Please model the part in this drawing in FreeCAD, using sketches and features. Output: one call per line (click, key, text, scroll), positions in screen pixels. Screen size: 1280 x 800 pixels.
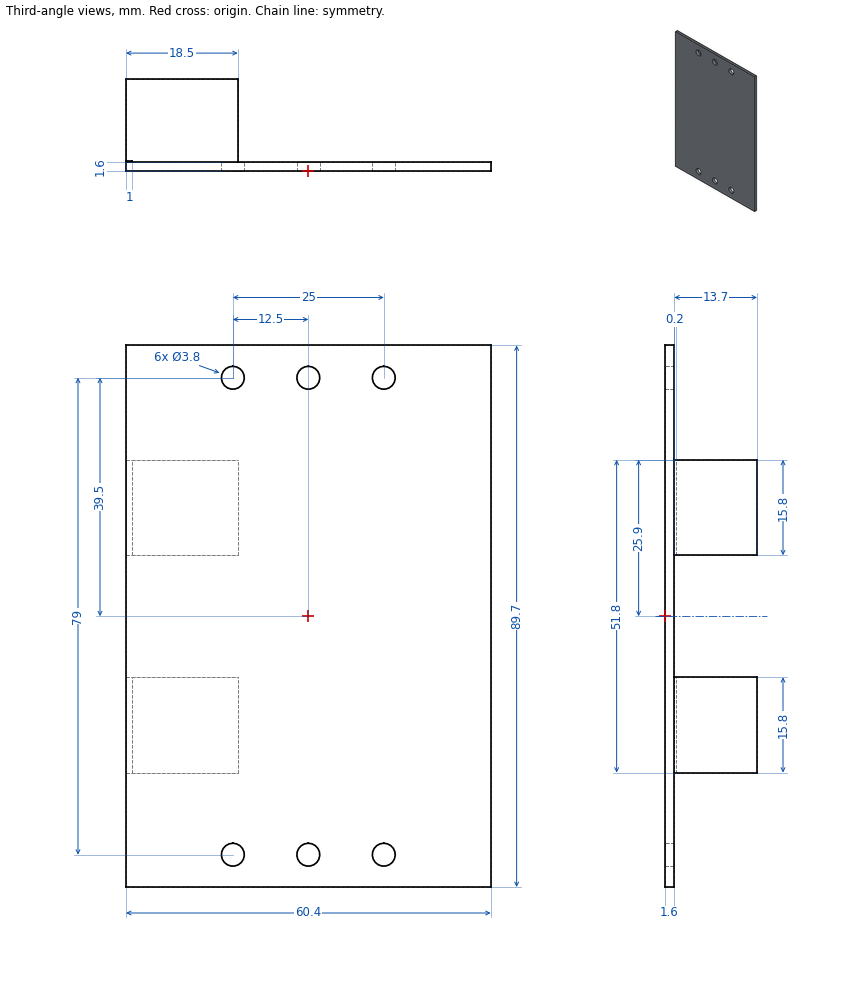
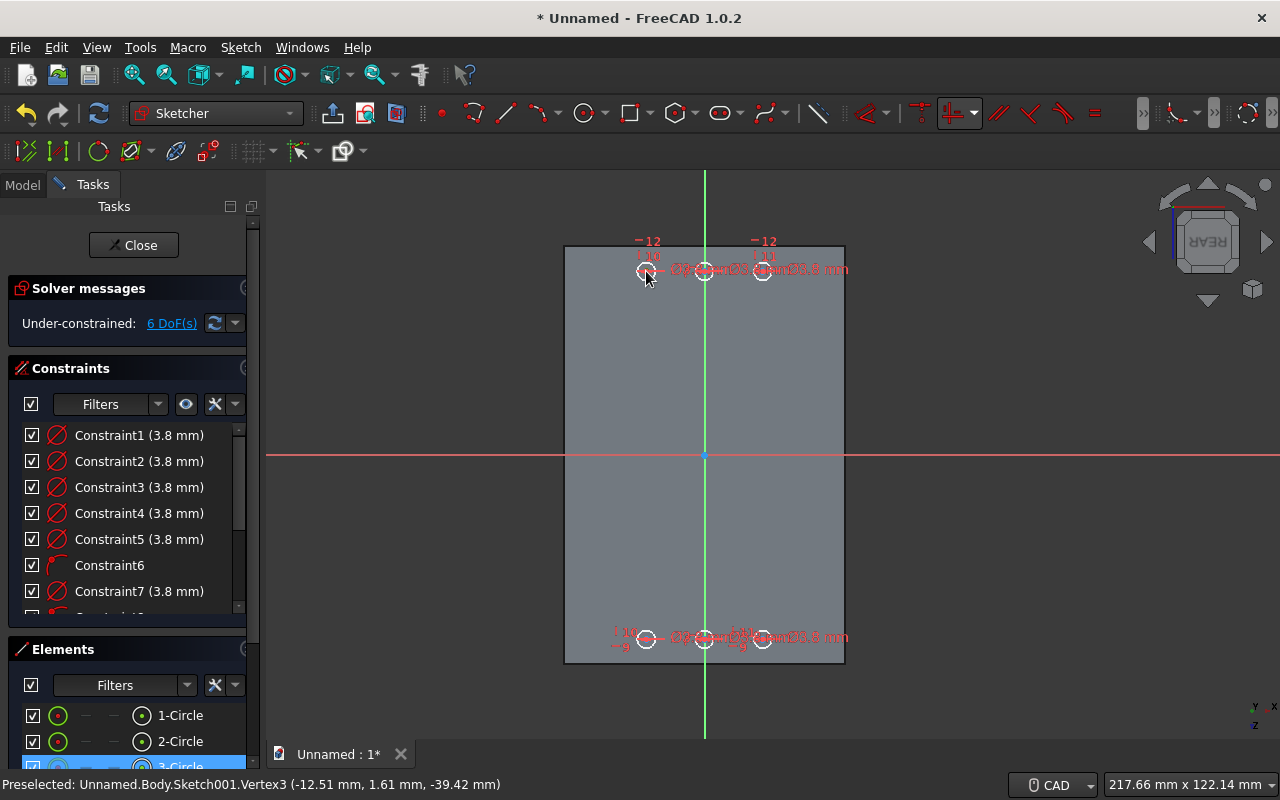
click(705, 271)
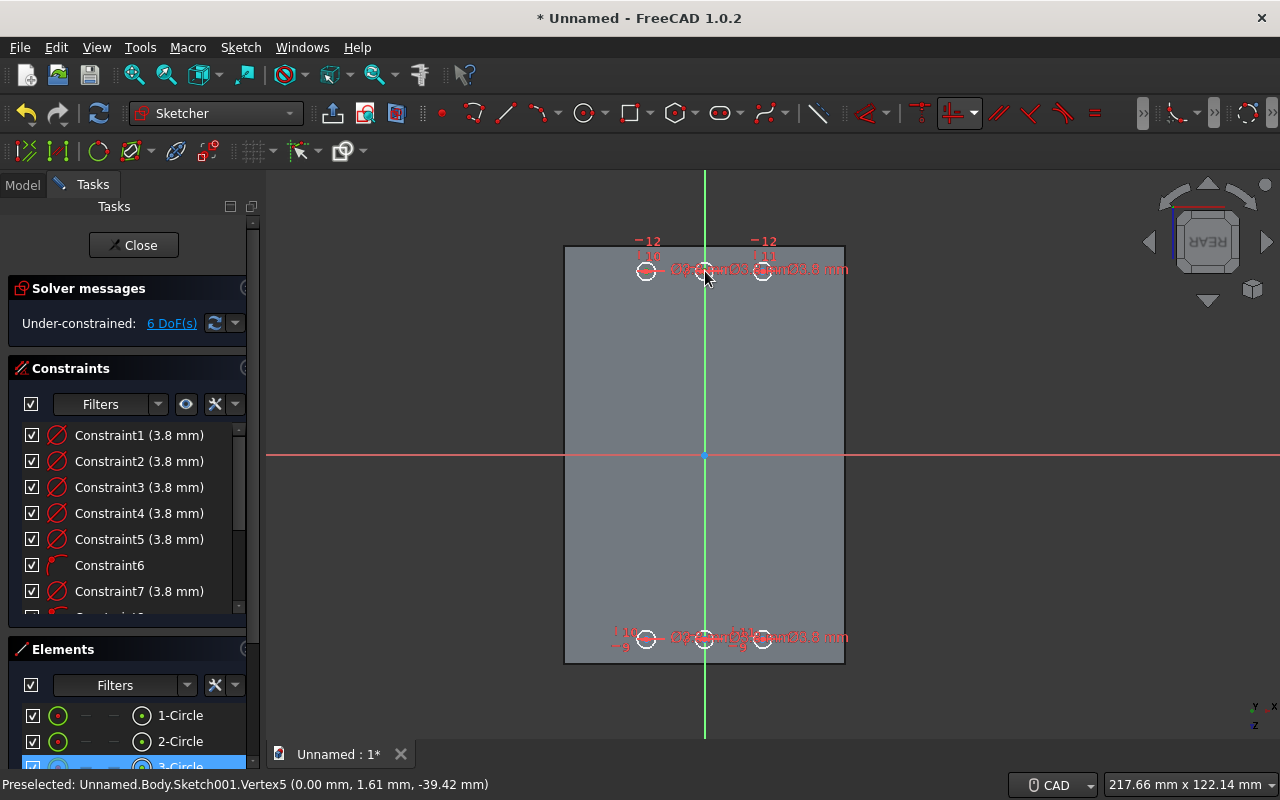
key(h)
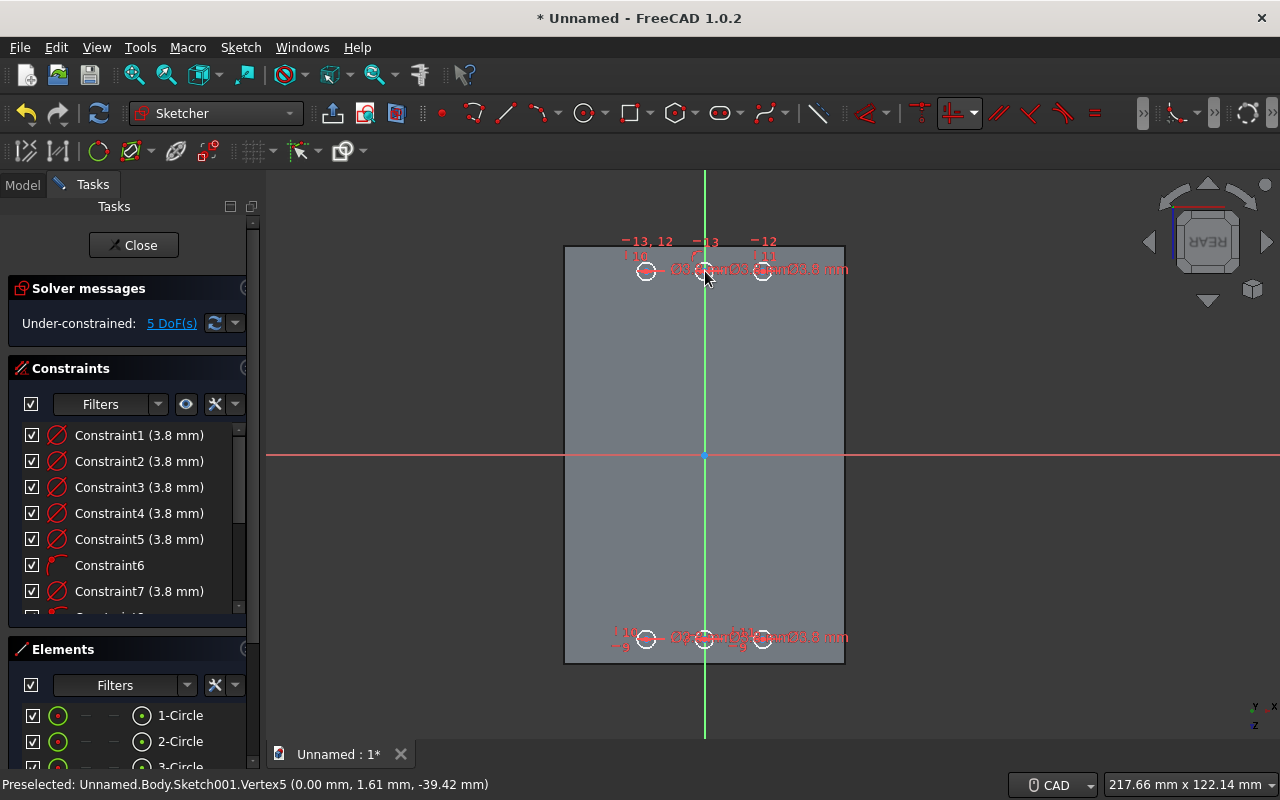
click(646, 639)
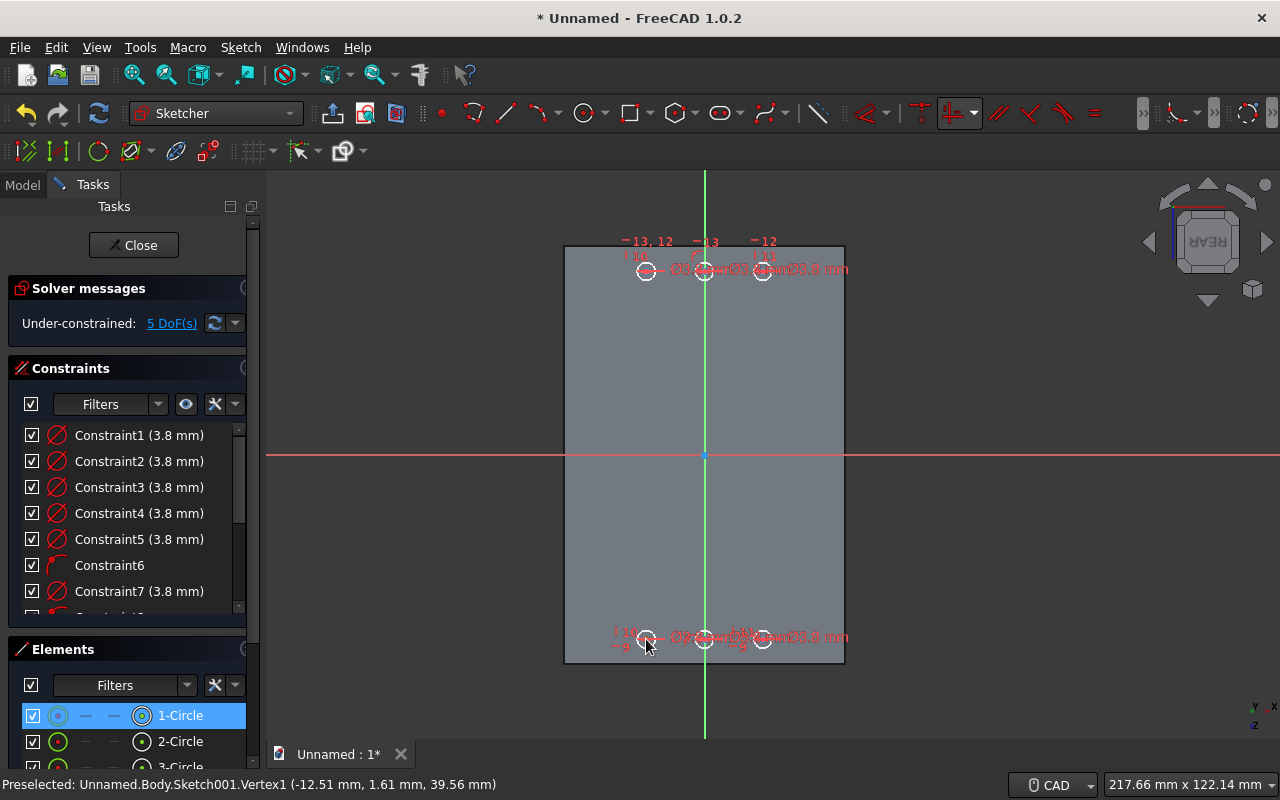
click(705, 639)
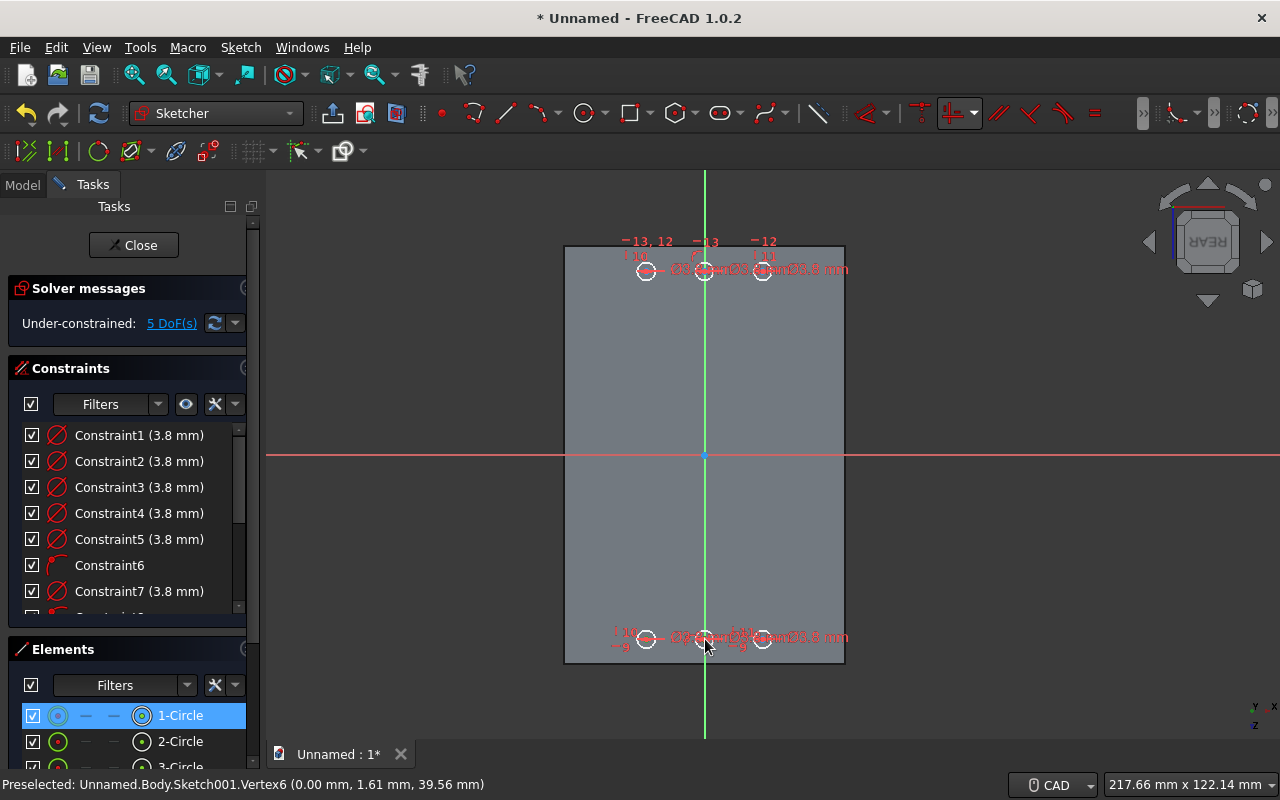
key(h)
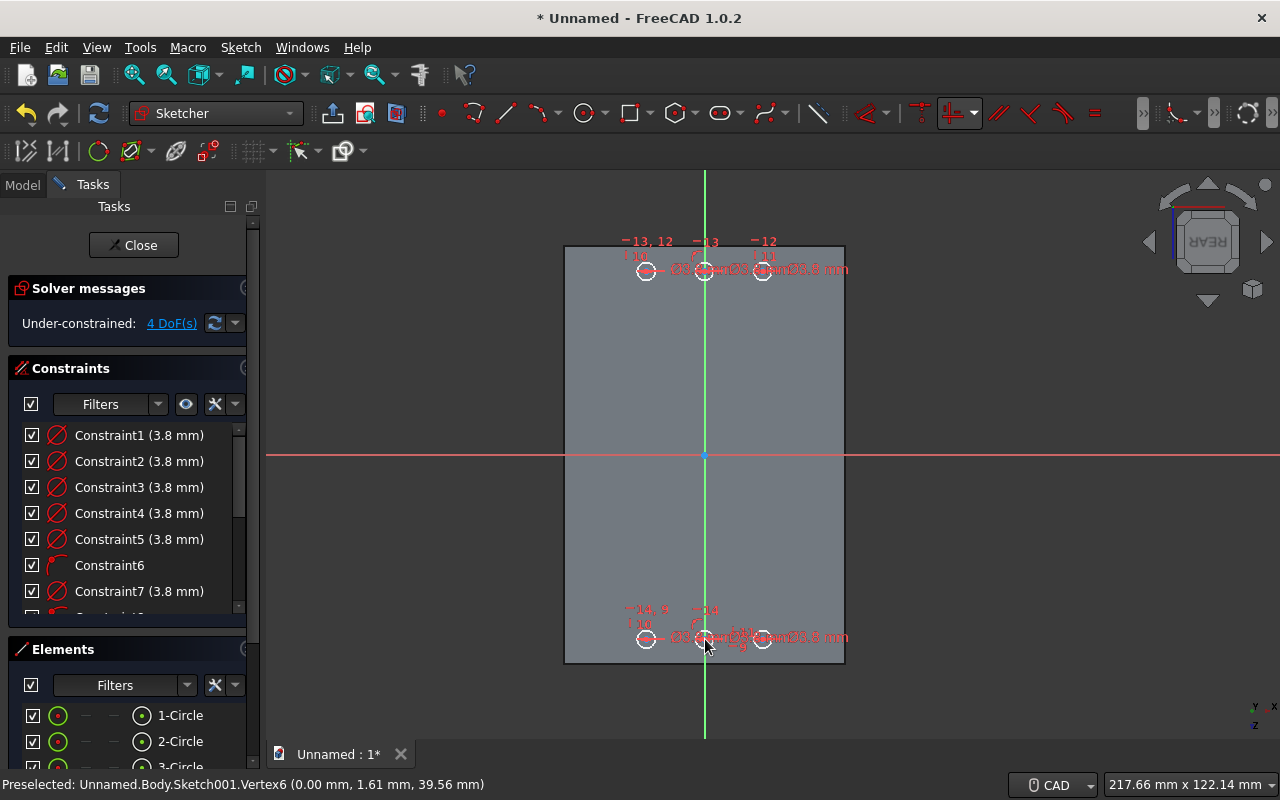
click(646, 639)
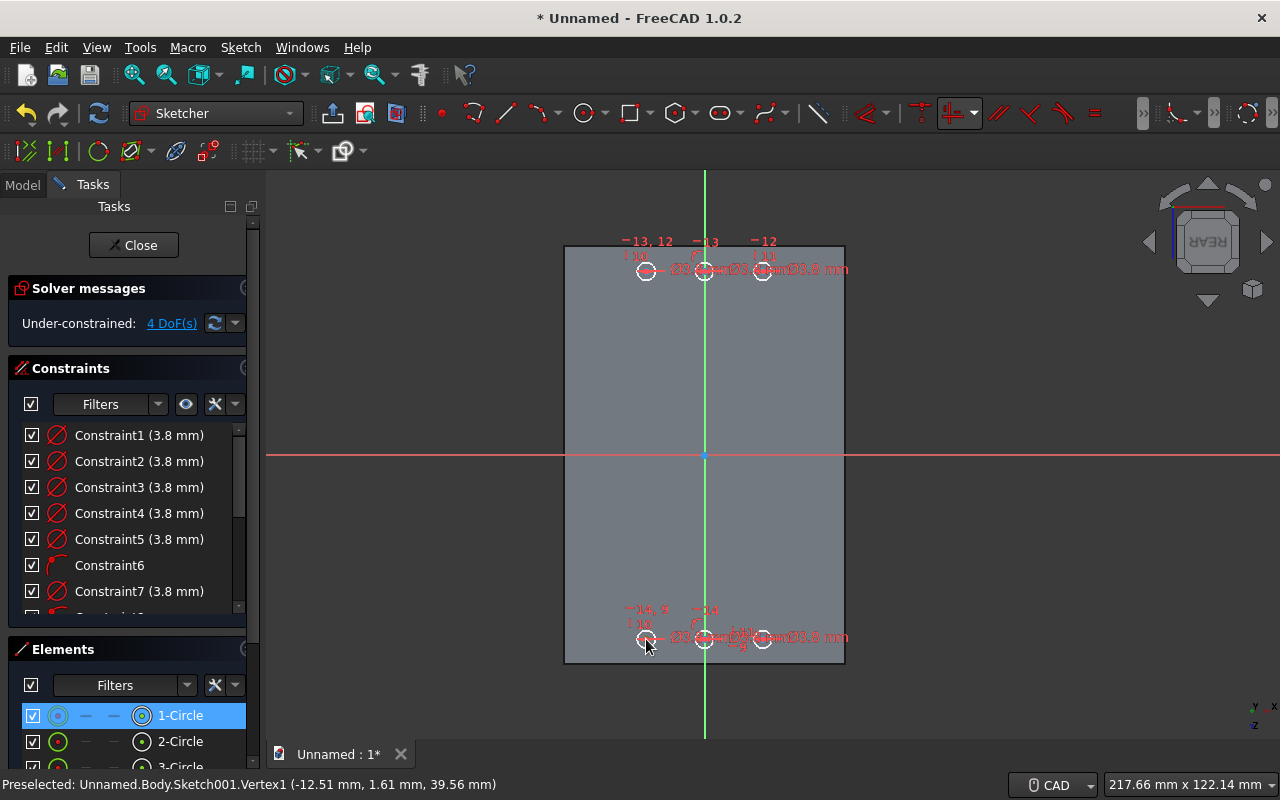
click(763, 639)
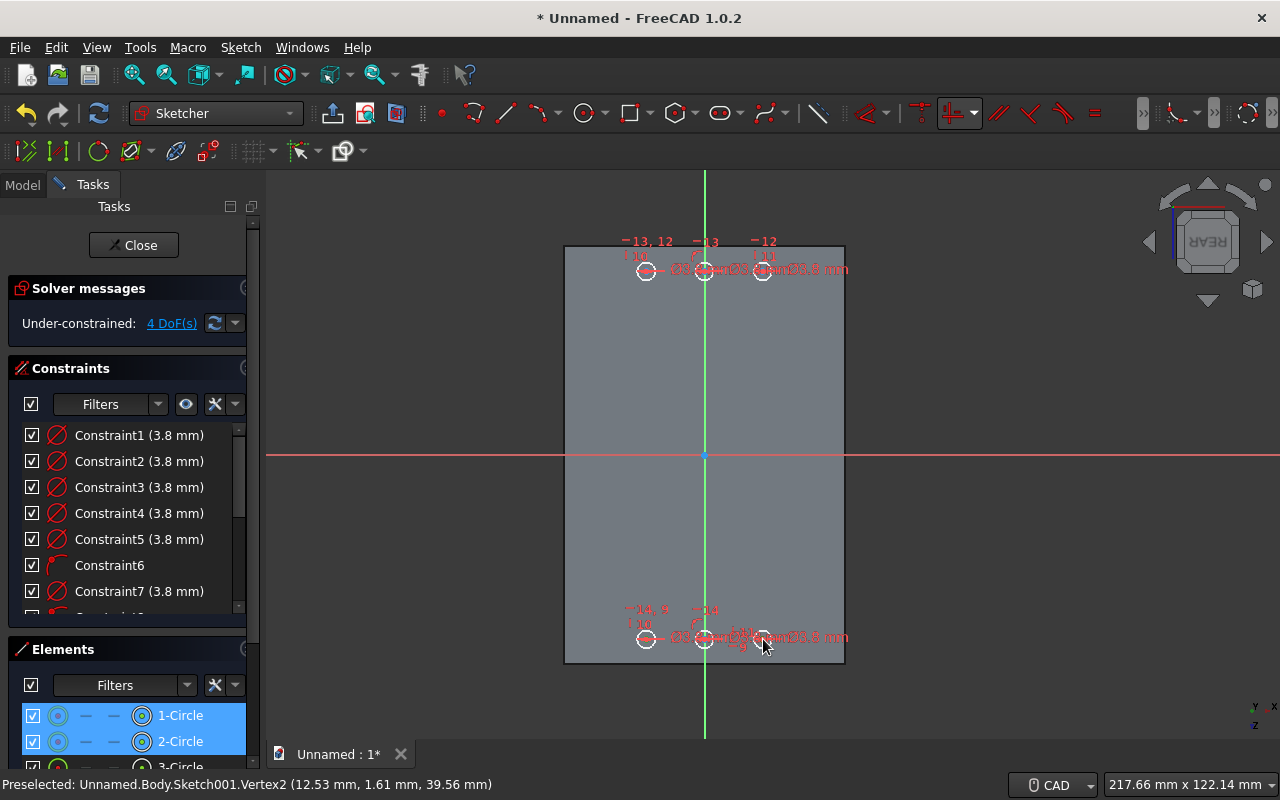
key(l)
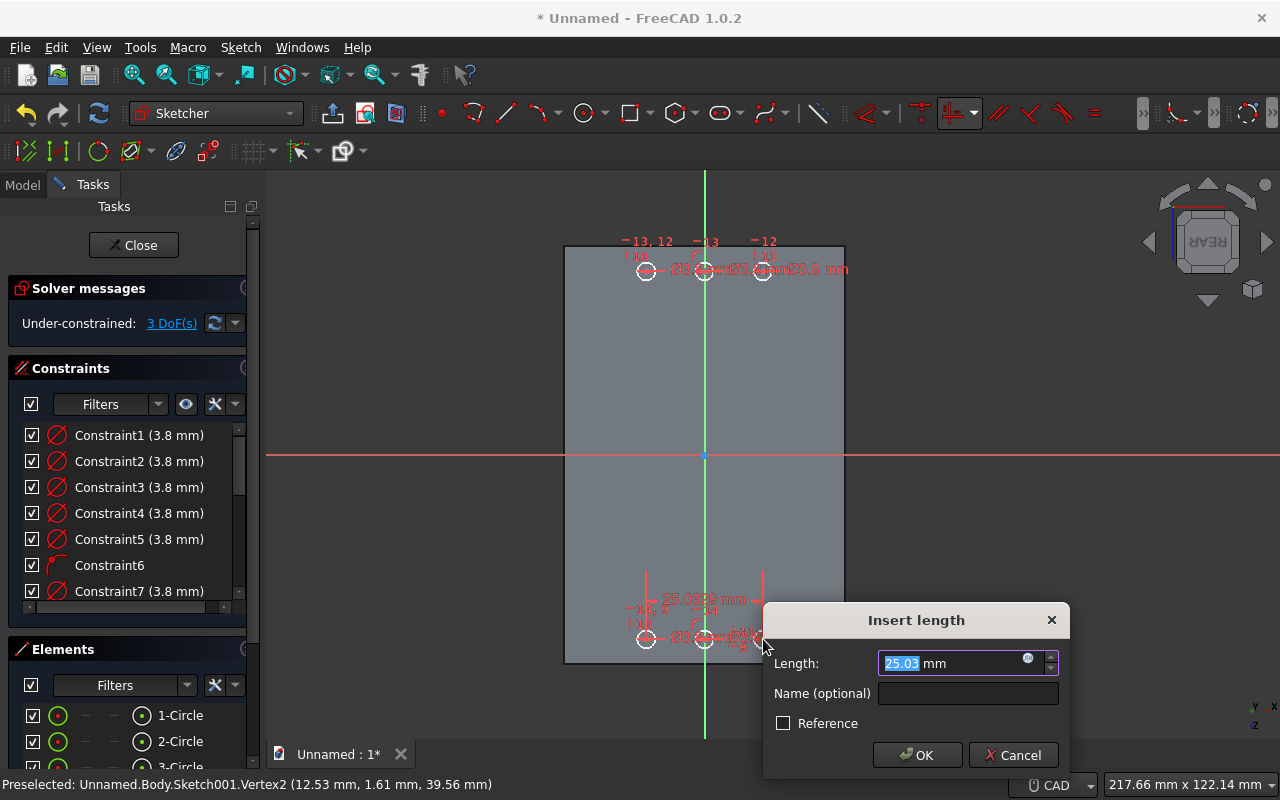
text(25)
key(Return)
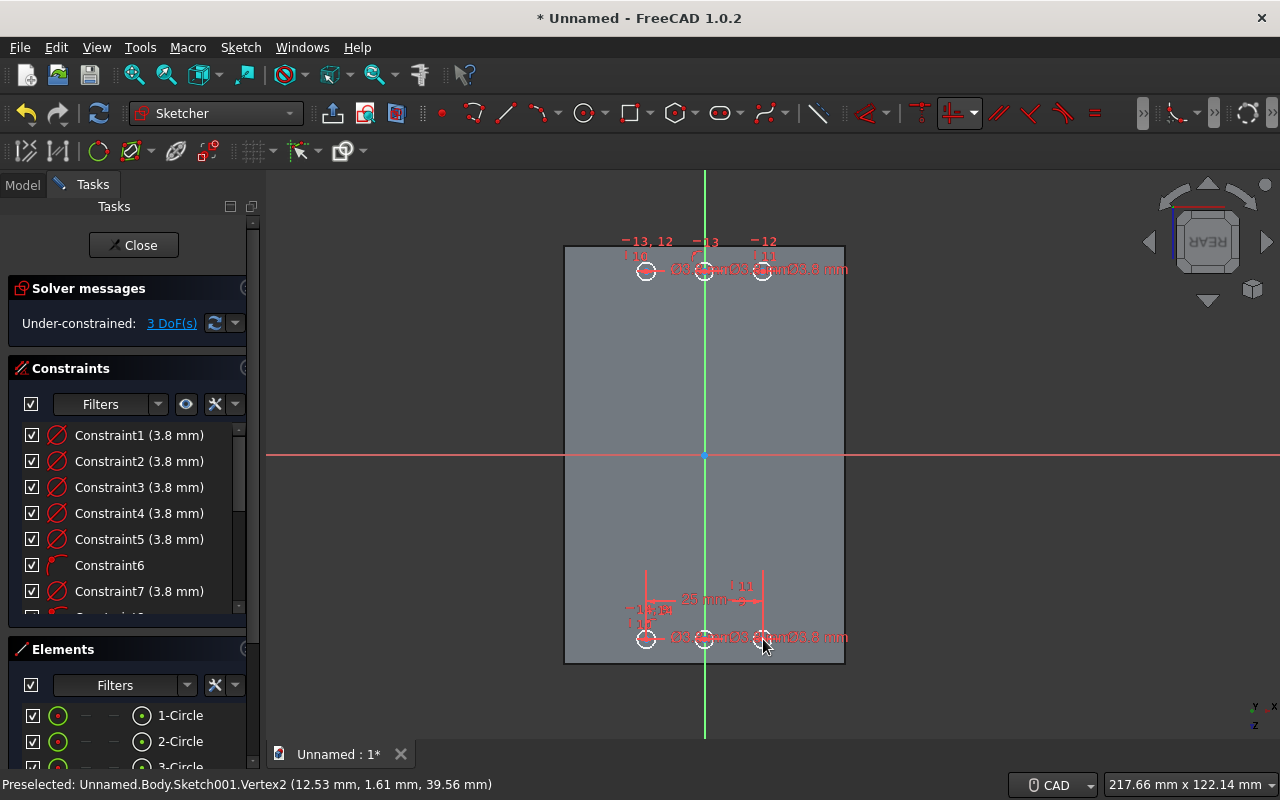
click(646, 639)